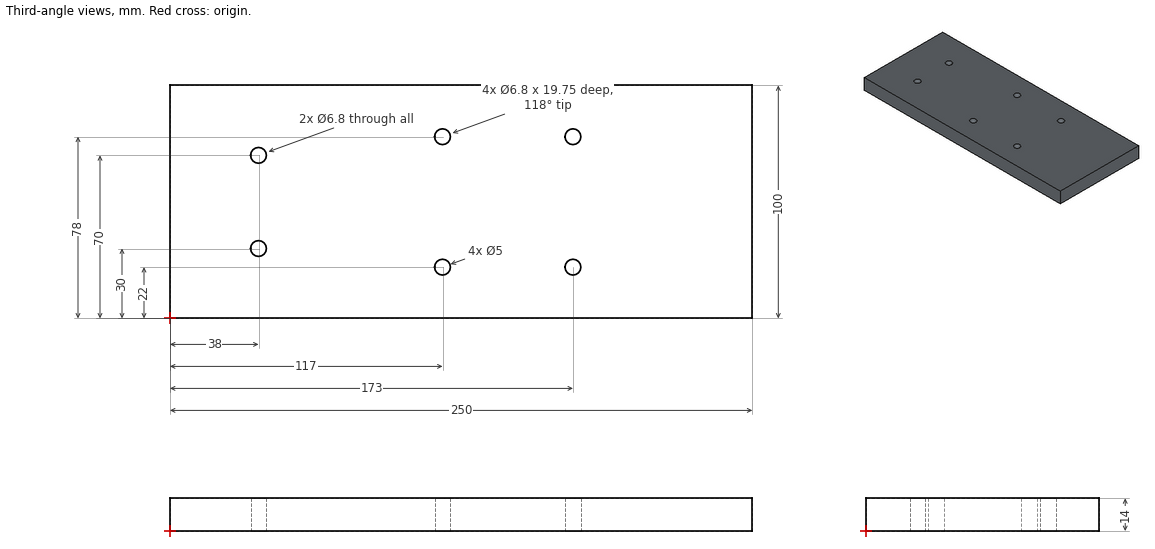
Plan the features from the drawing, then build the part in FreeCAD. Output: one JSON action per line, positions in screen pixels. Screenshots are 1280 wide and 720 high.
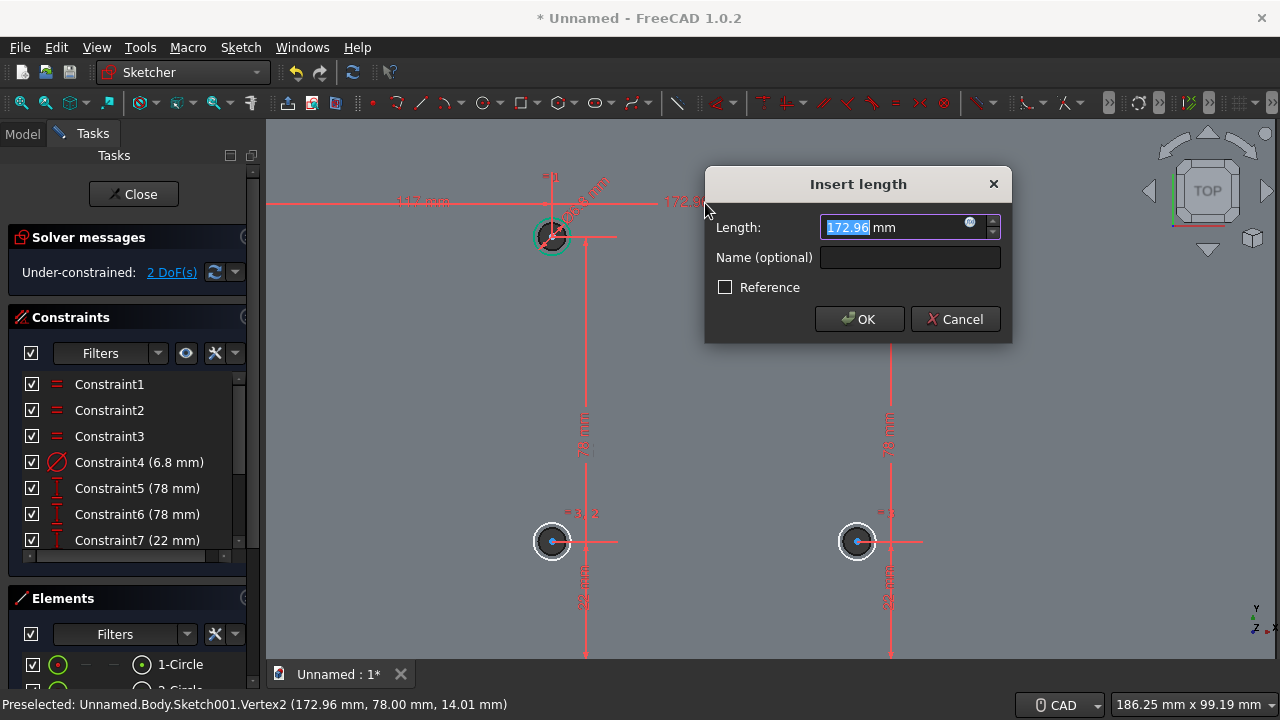
{"action": "type", "text": "173"}
{"action": "key", "text": "Return"}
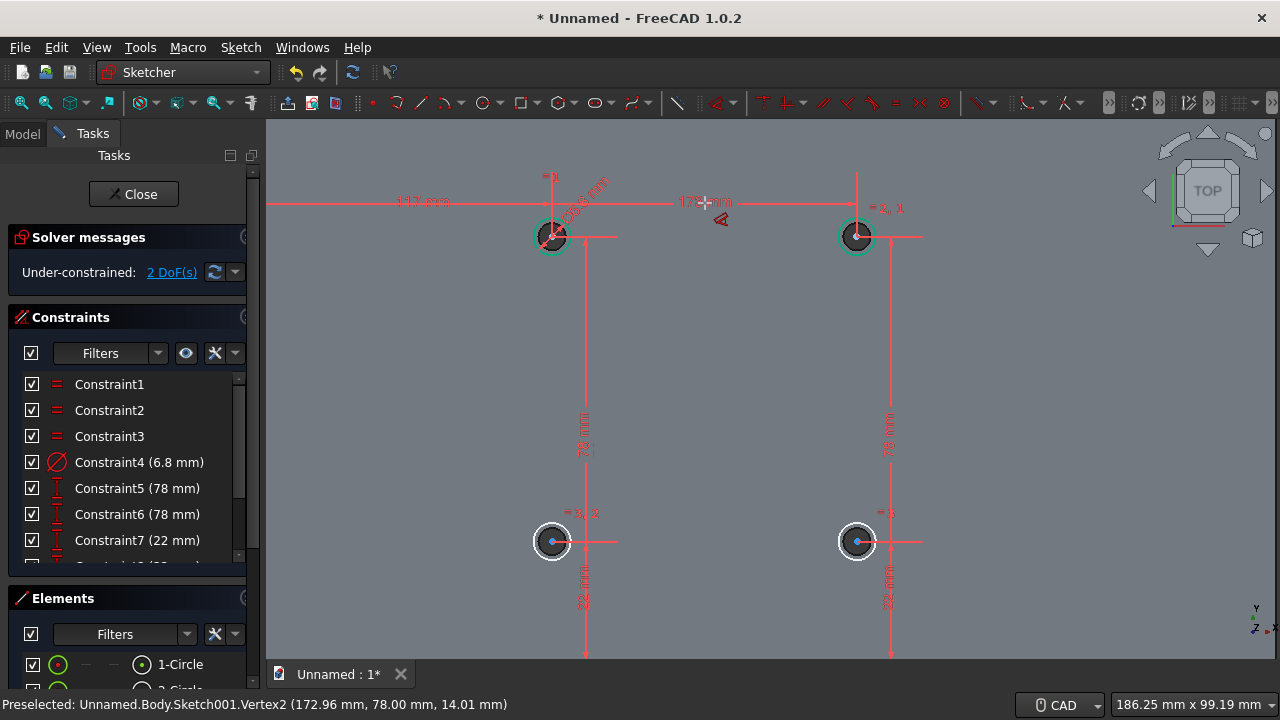
{"action": "left_click", "coordinate": [552, 542]}
{"action": "left_click", "coordinate": [423, 508]}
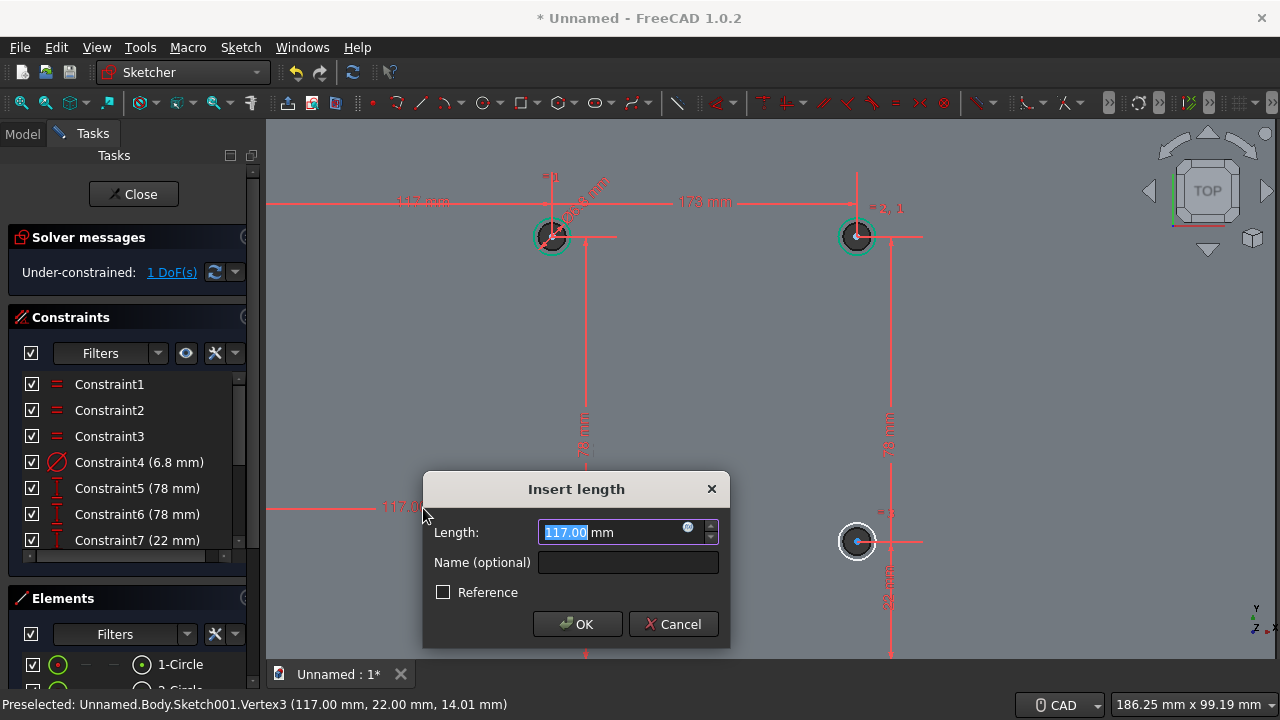
{"action": "type", "text": "117"}
{"action": "key", "text": "Return"}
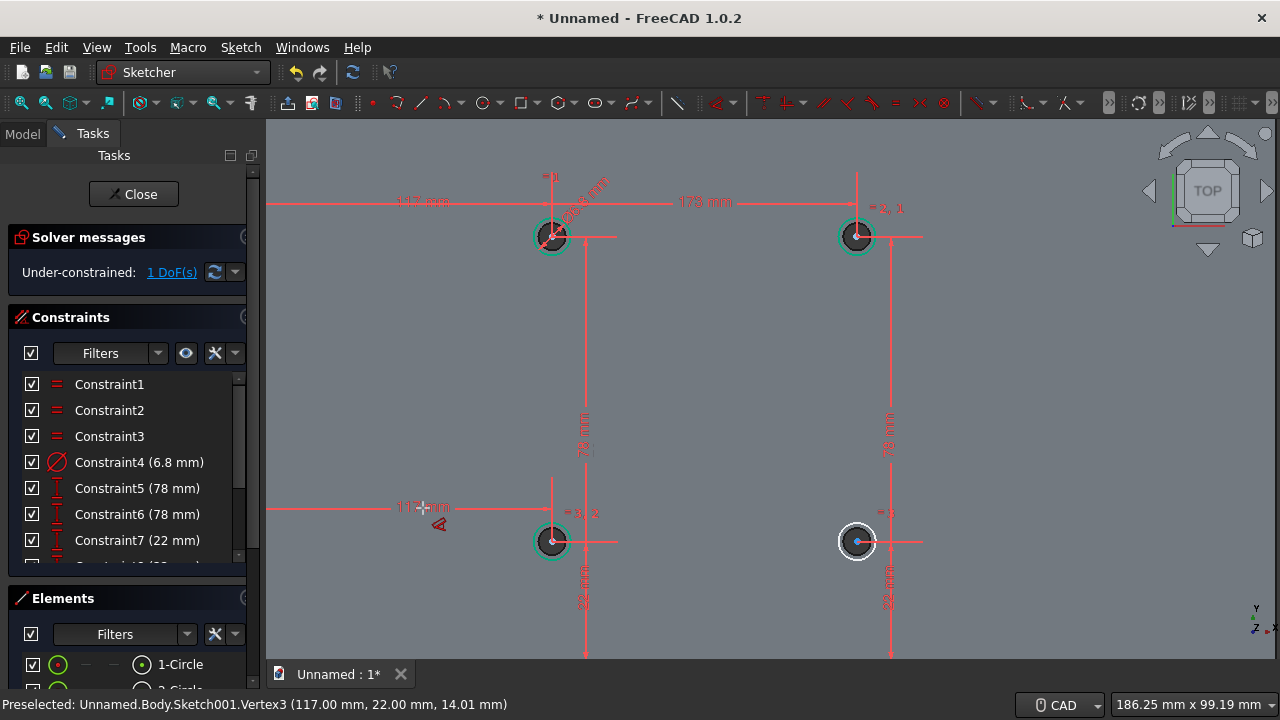
{"action": "left_click", "coordinate": [857, 542]}
{"action": "left_click", "coordinate": [576, 508]}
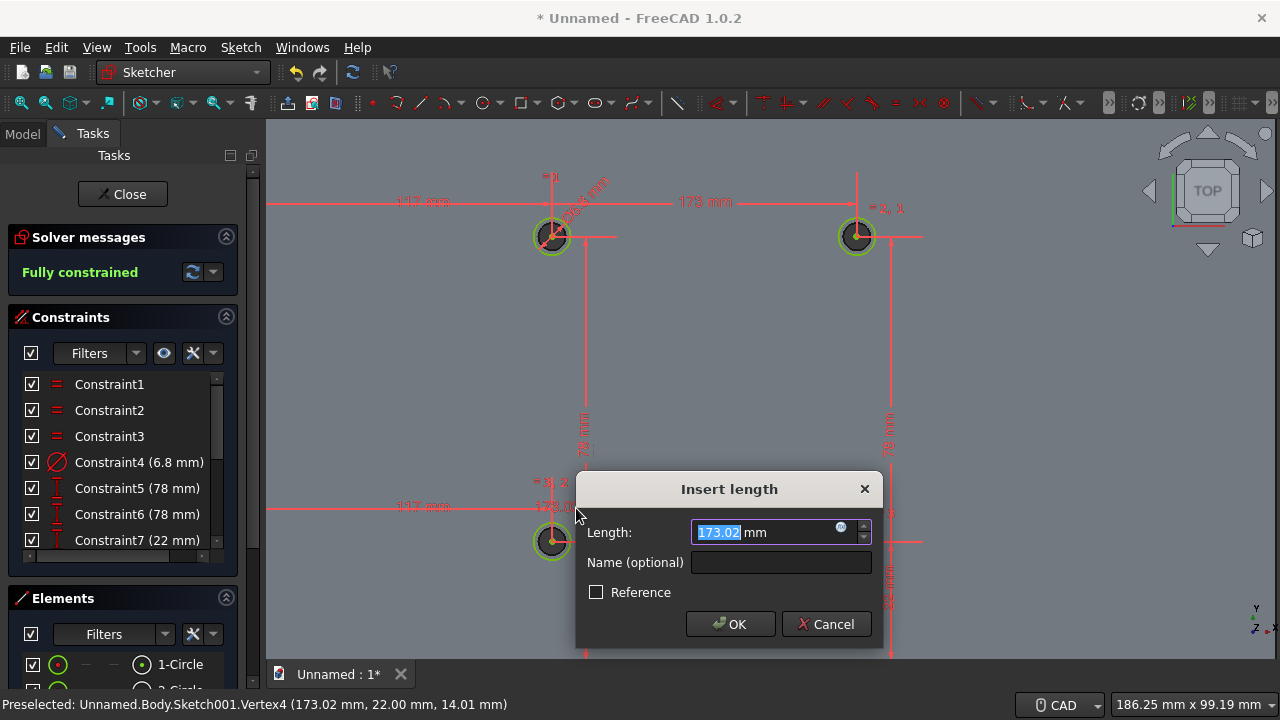
{"action": "type", "text": "173"}
{"action": "key", "text": "Return"}
{"action": "key", "text": "Escape"}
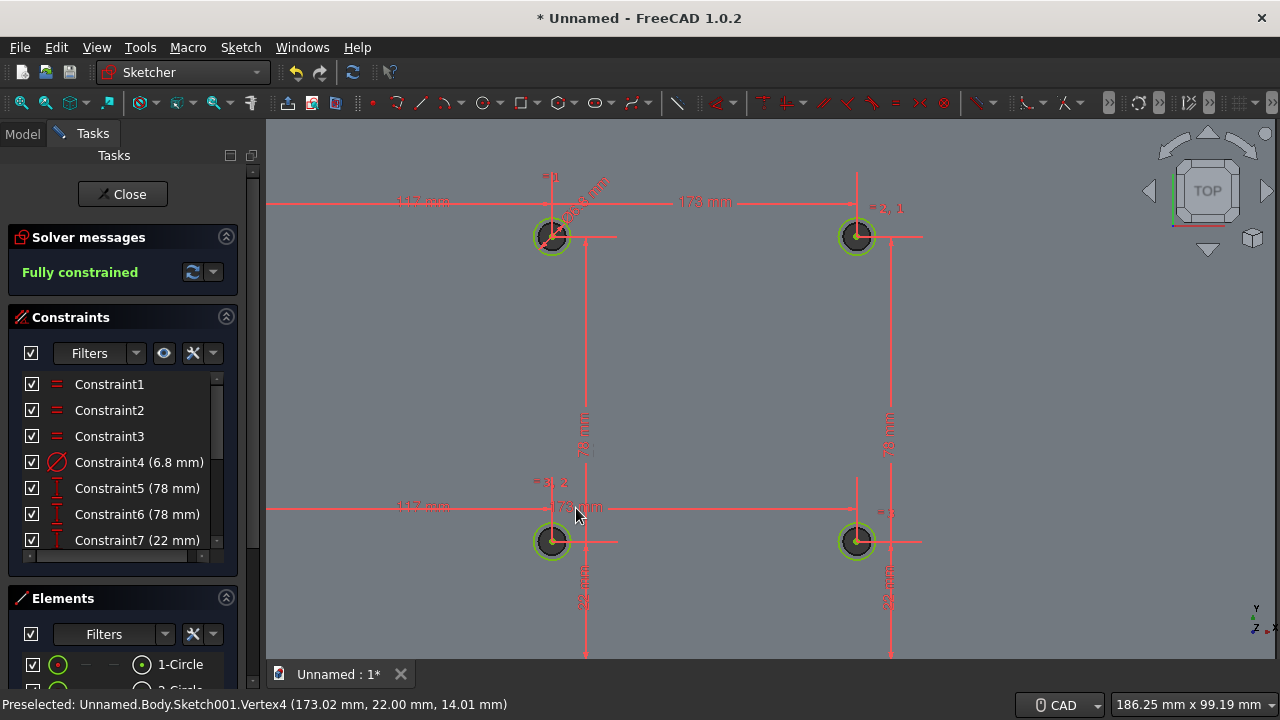
{"action": "left_click", "coordinate": [123, 194]}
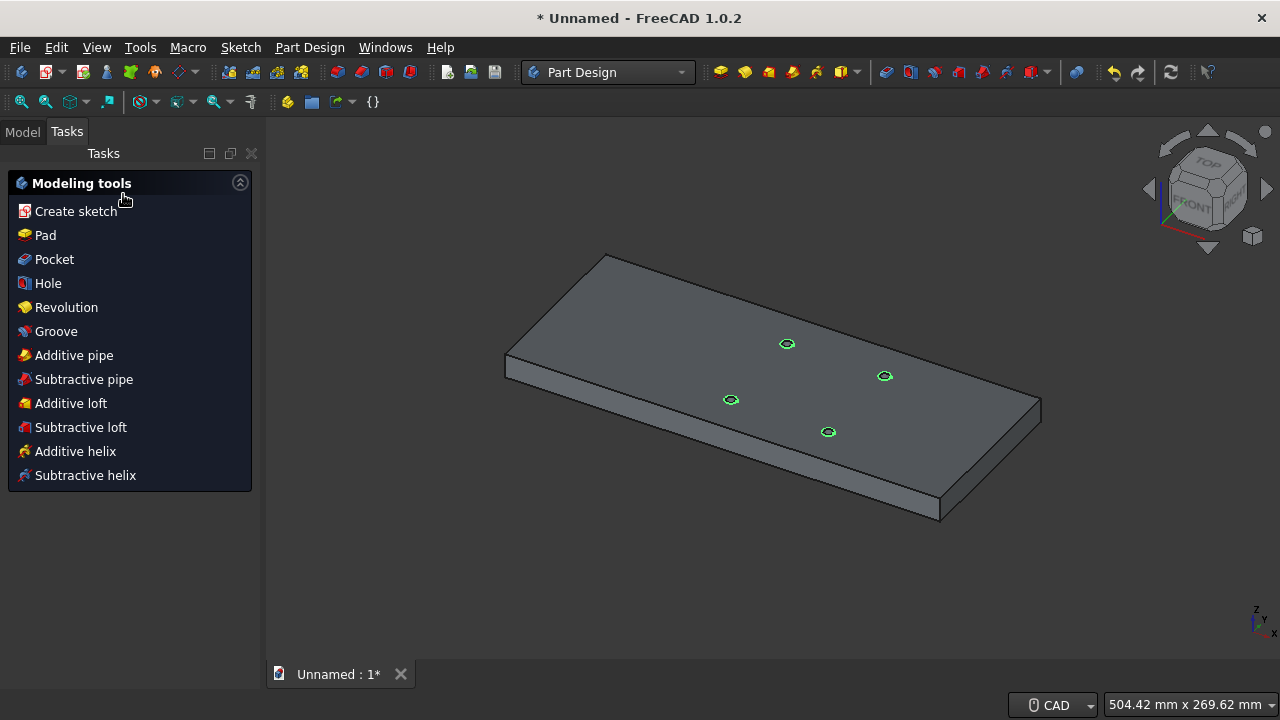
{"action": "left_click", "coordinate": [912, 72]}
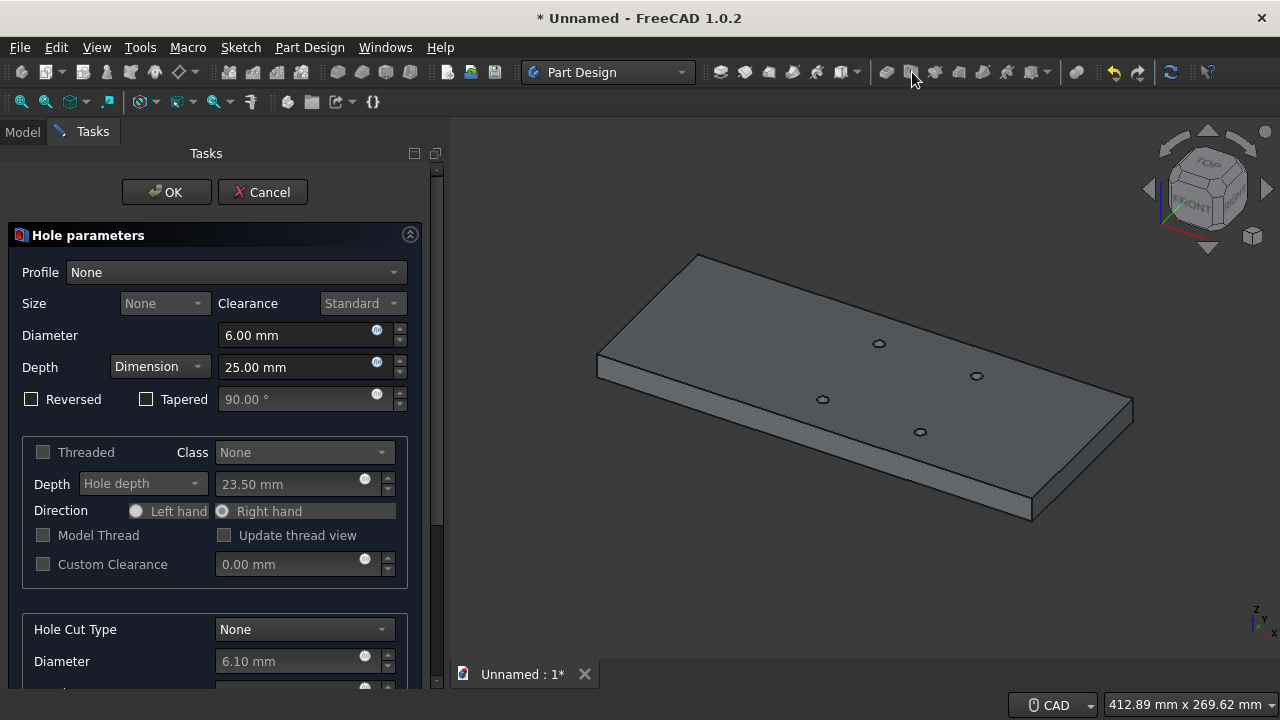
{"action": "triple_click", "coordinate": [305, 335]}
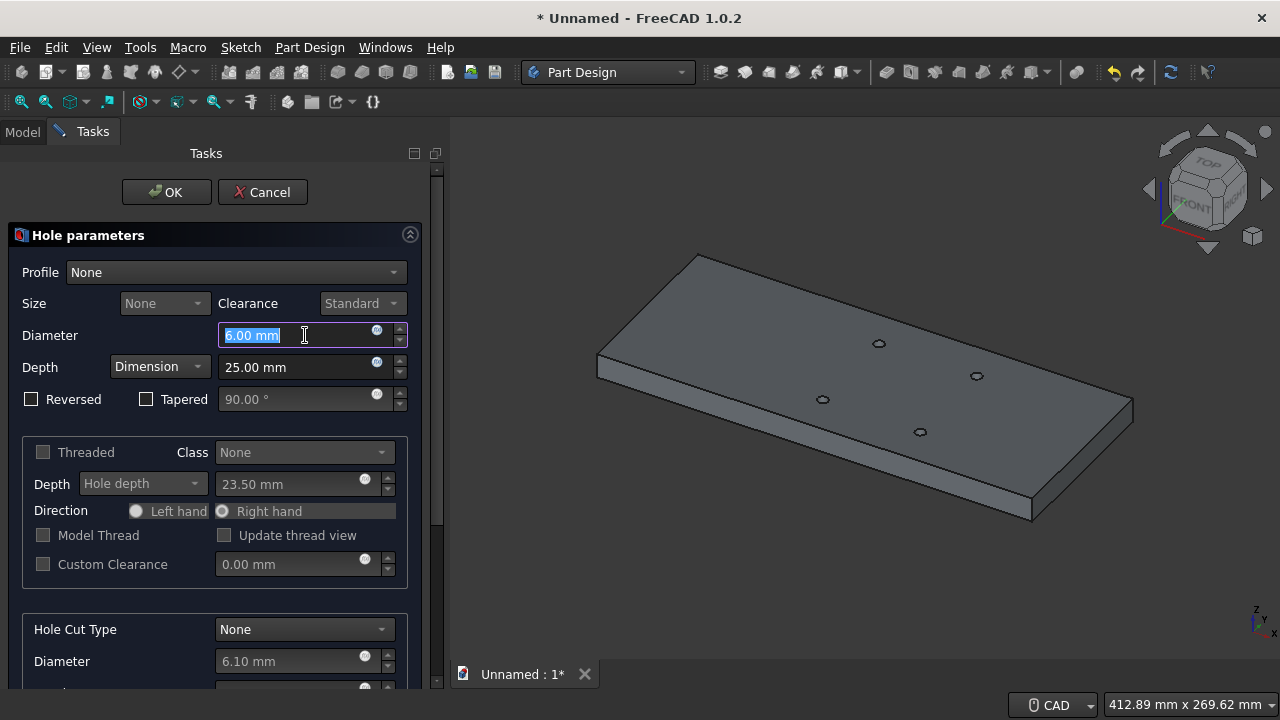
{"action": "type", "text": "6.8"}
{"action": "key", "text": "Tab"}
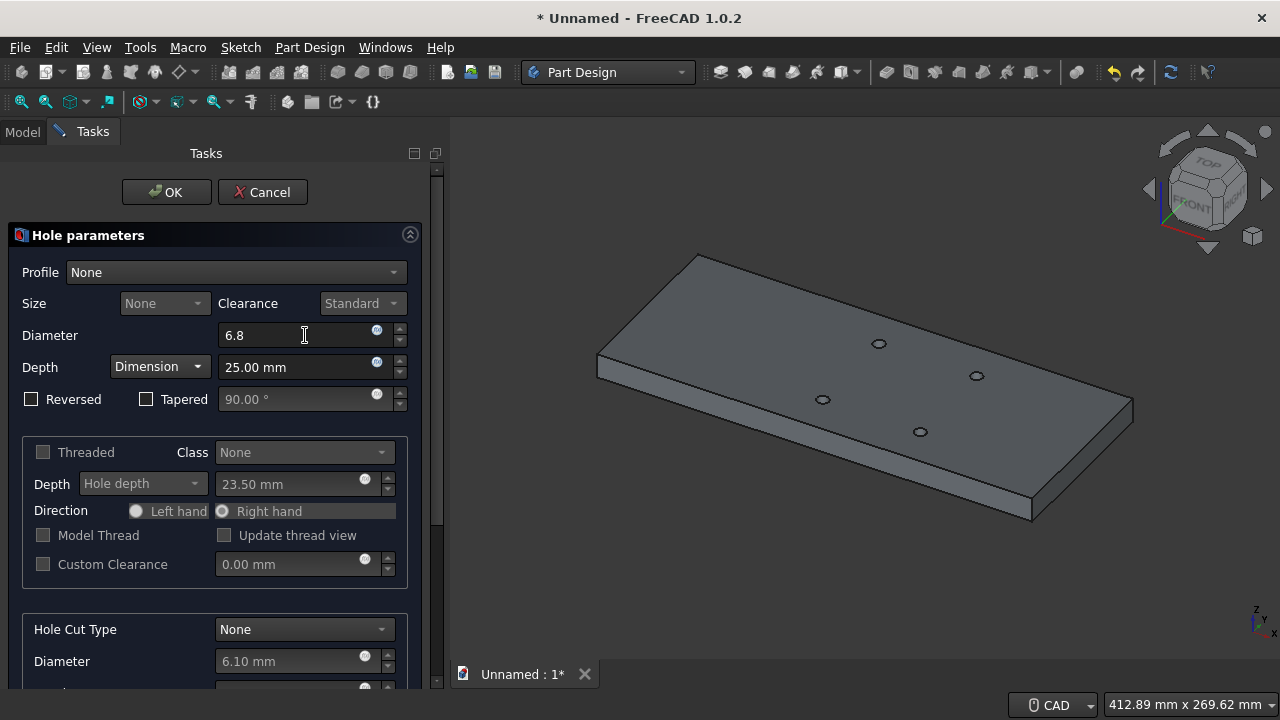
{"action": "triple_click", "coordinate": [305, 367]}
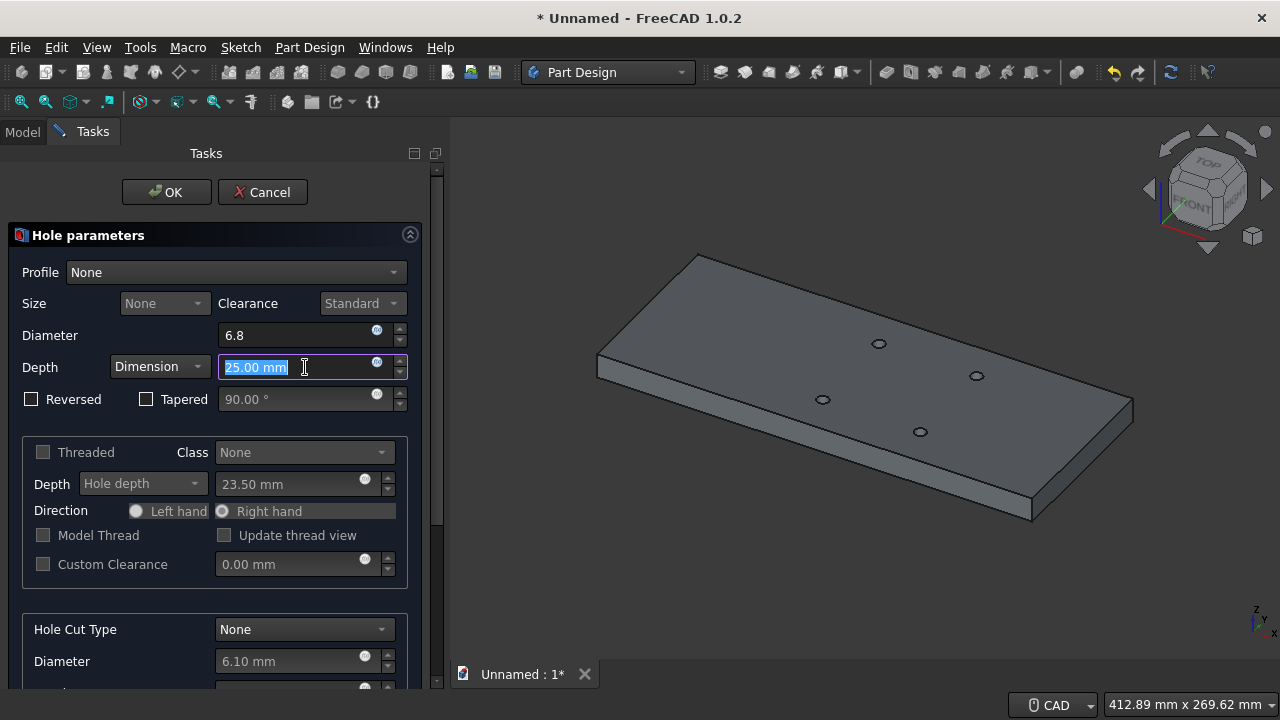
{"action": "type", "text": "19.75"}
{"action": "key", "text": "Tab"}